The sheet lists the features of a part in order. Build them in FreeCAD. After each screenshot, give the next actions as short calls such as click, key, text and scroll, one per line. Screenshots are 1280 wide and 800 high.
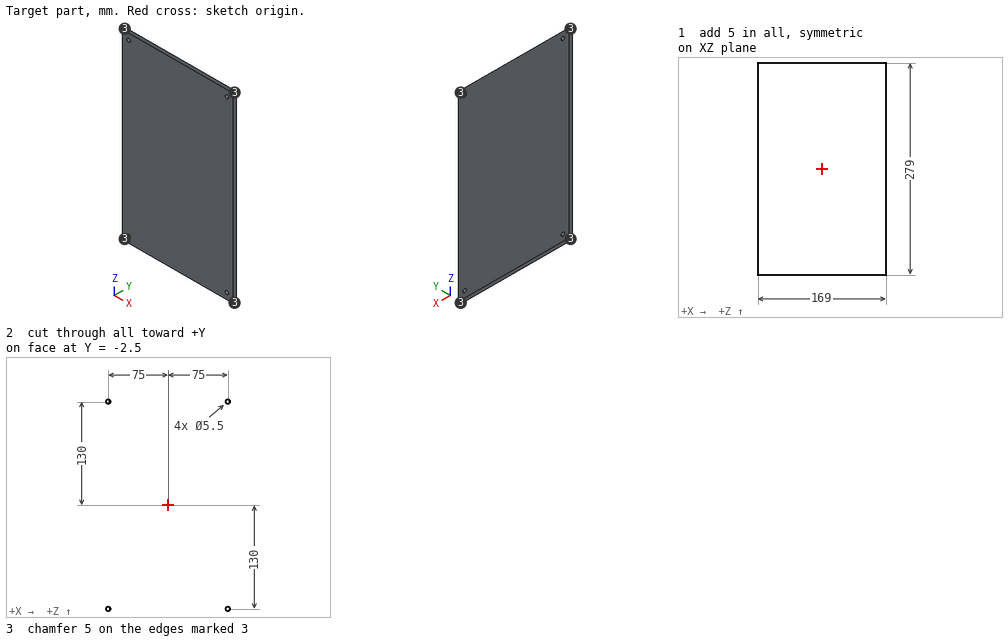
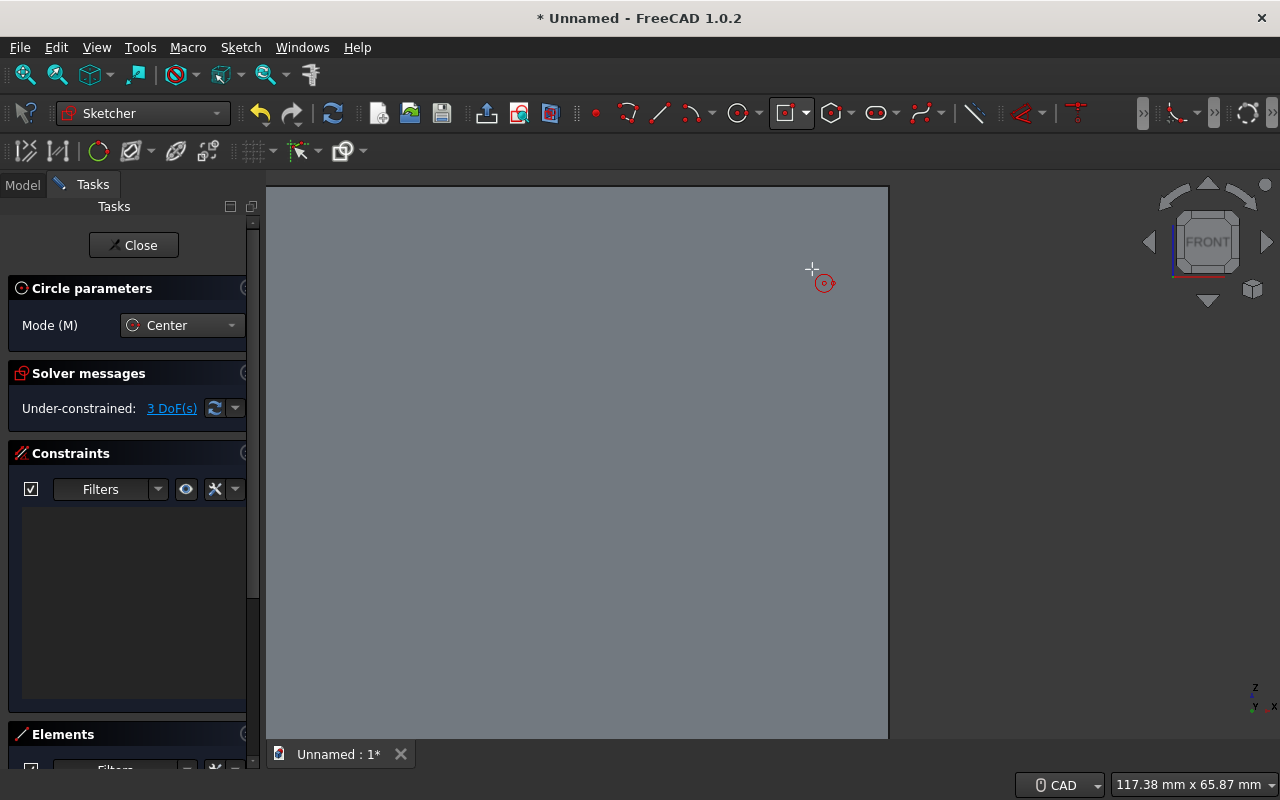
scroll(813, 269, down, 9)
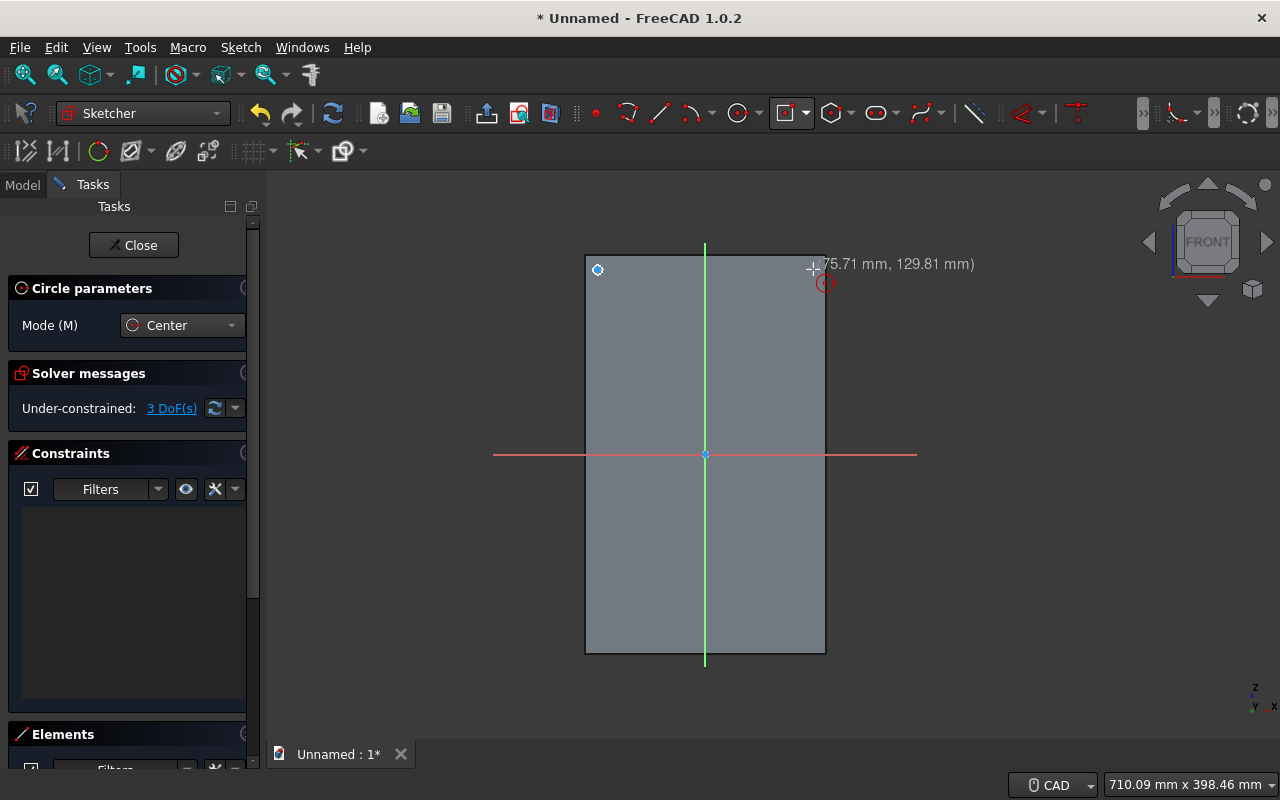
click(812, 269)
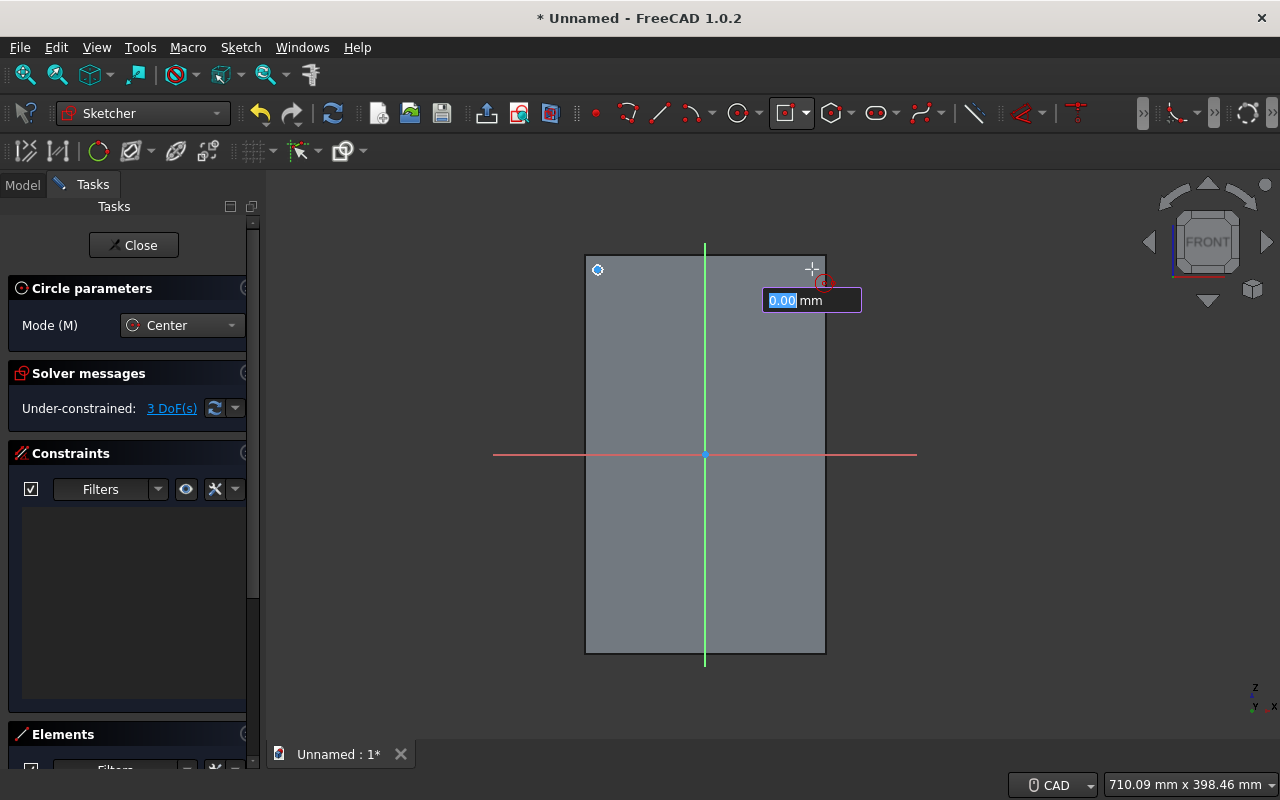
scroll(815, 266, up, 7)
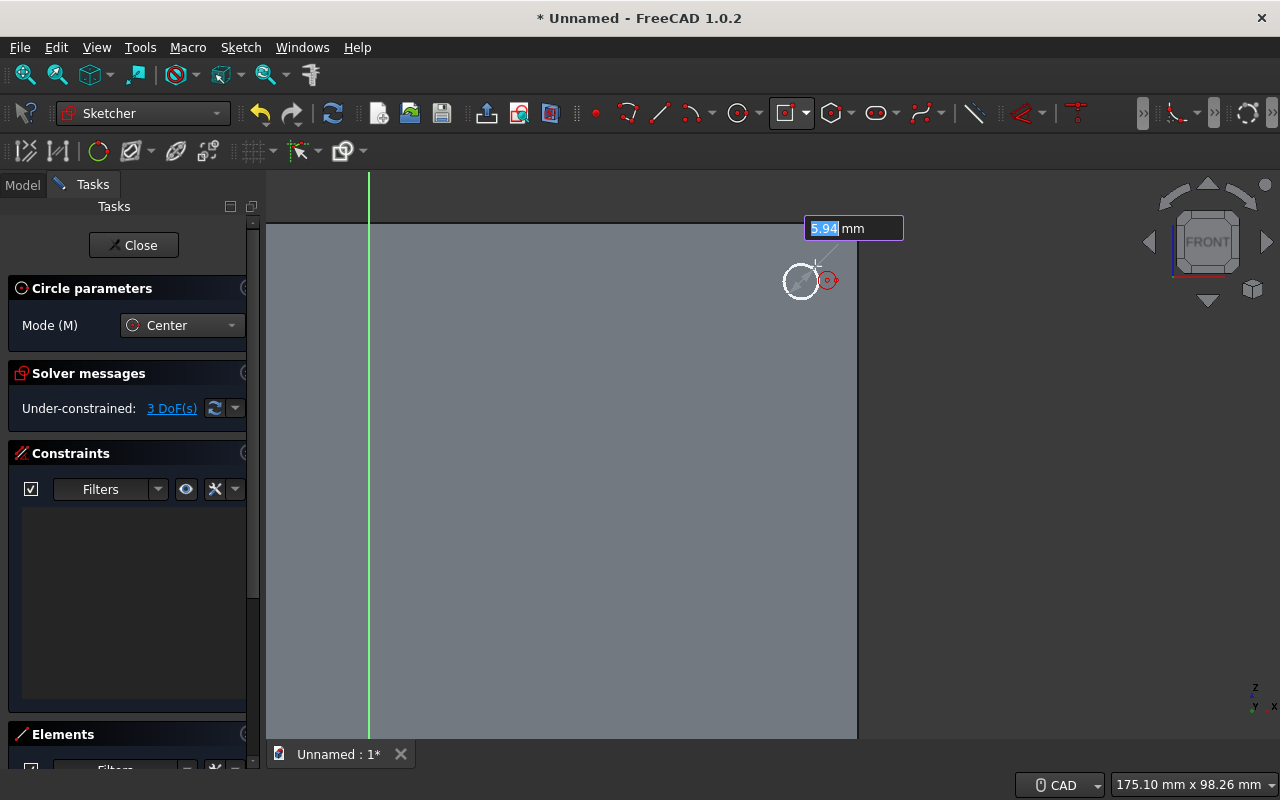
click(814, 267)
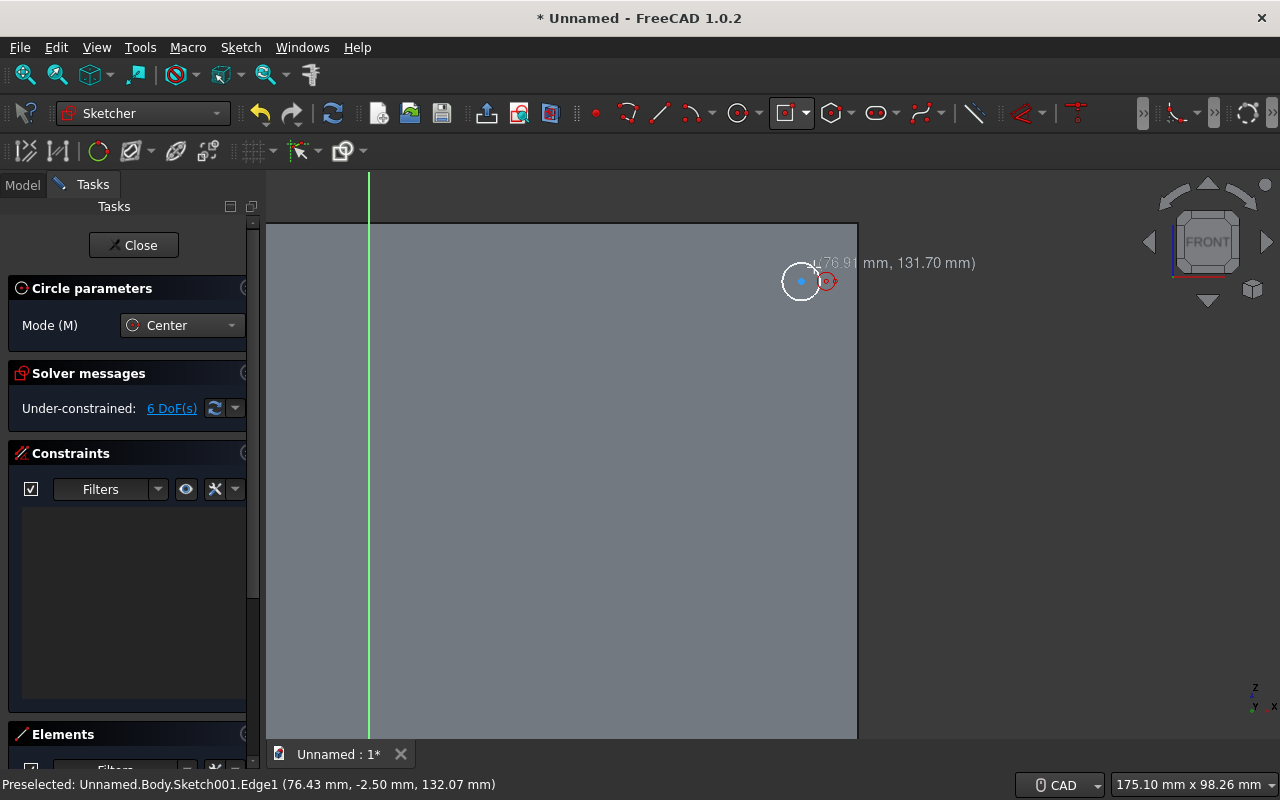
scroll(814, 266, down, 7)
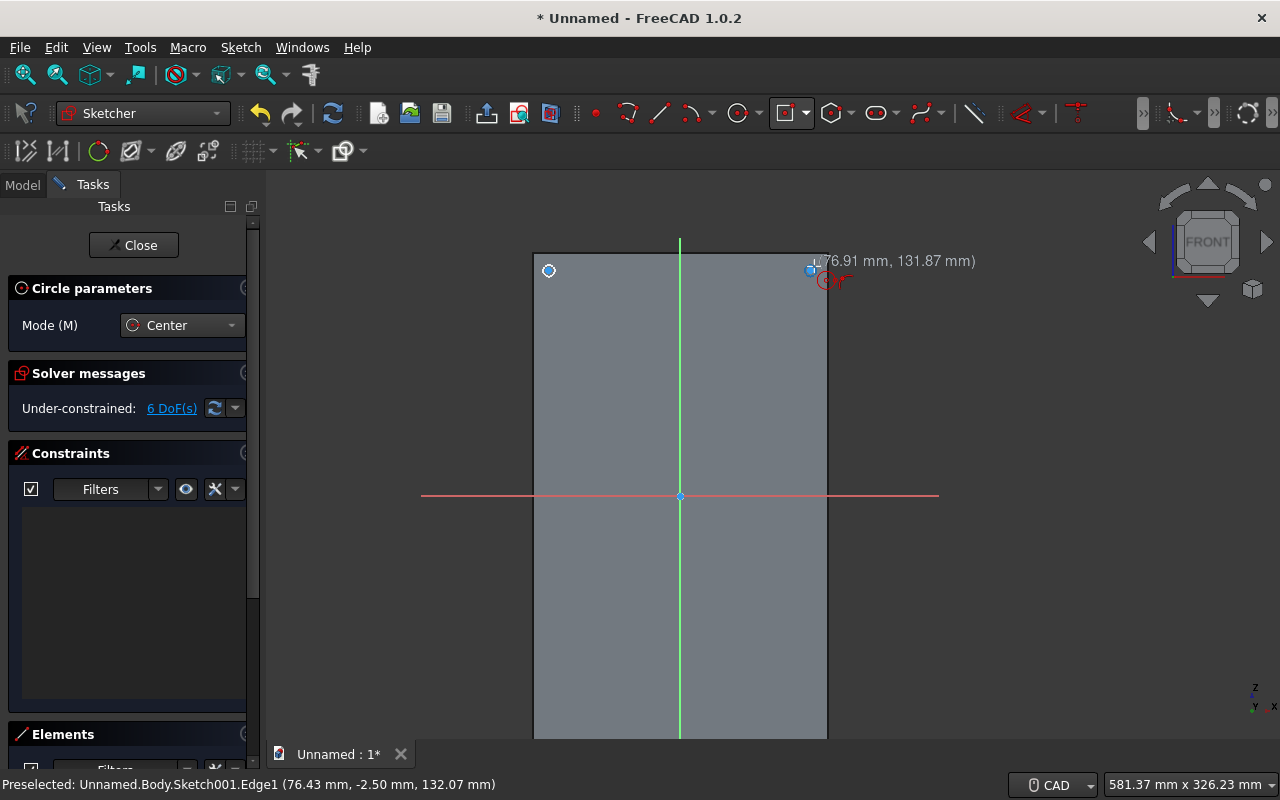
scroll(812, 640, up, 9)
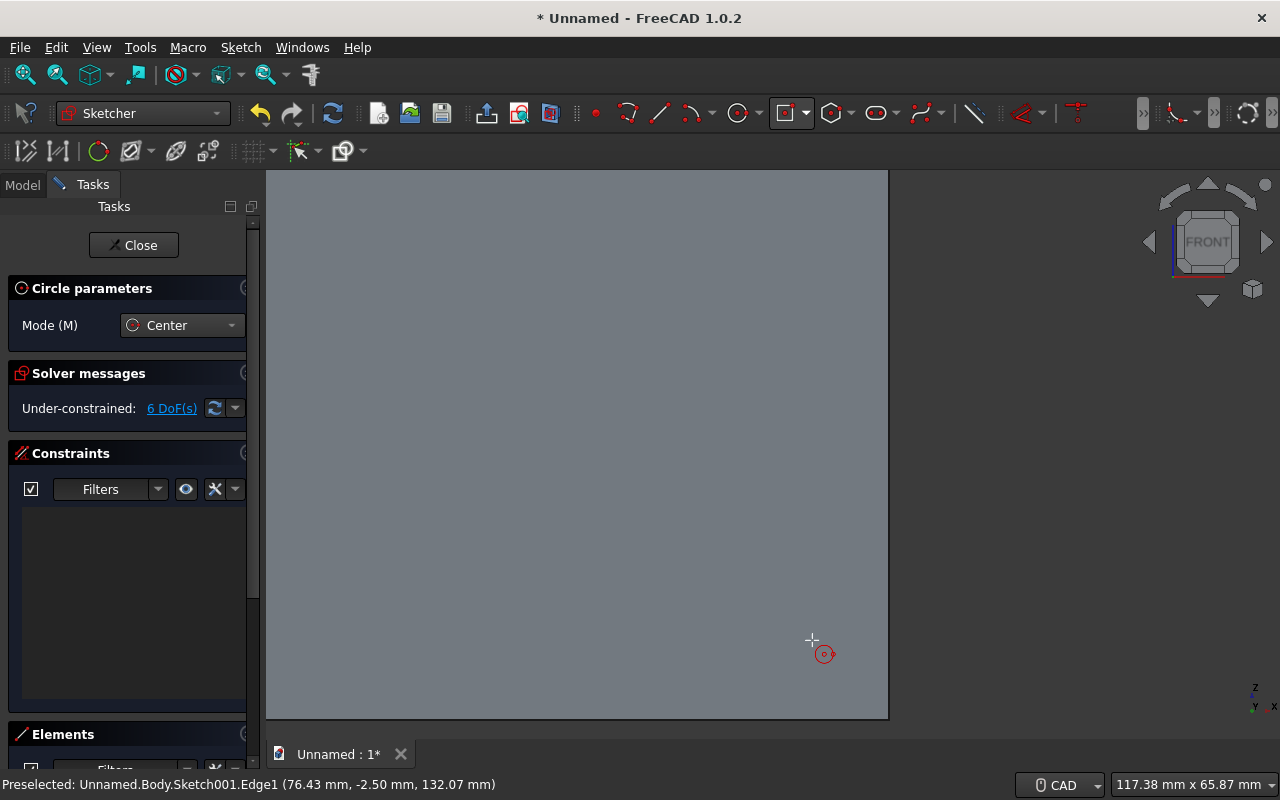
scroll(812, 641, down, 9)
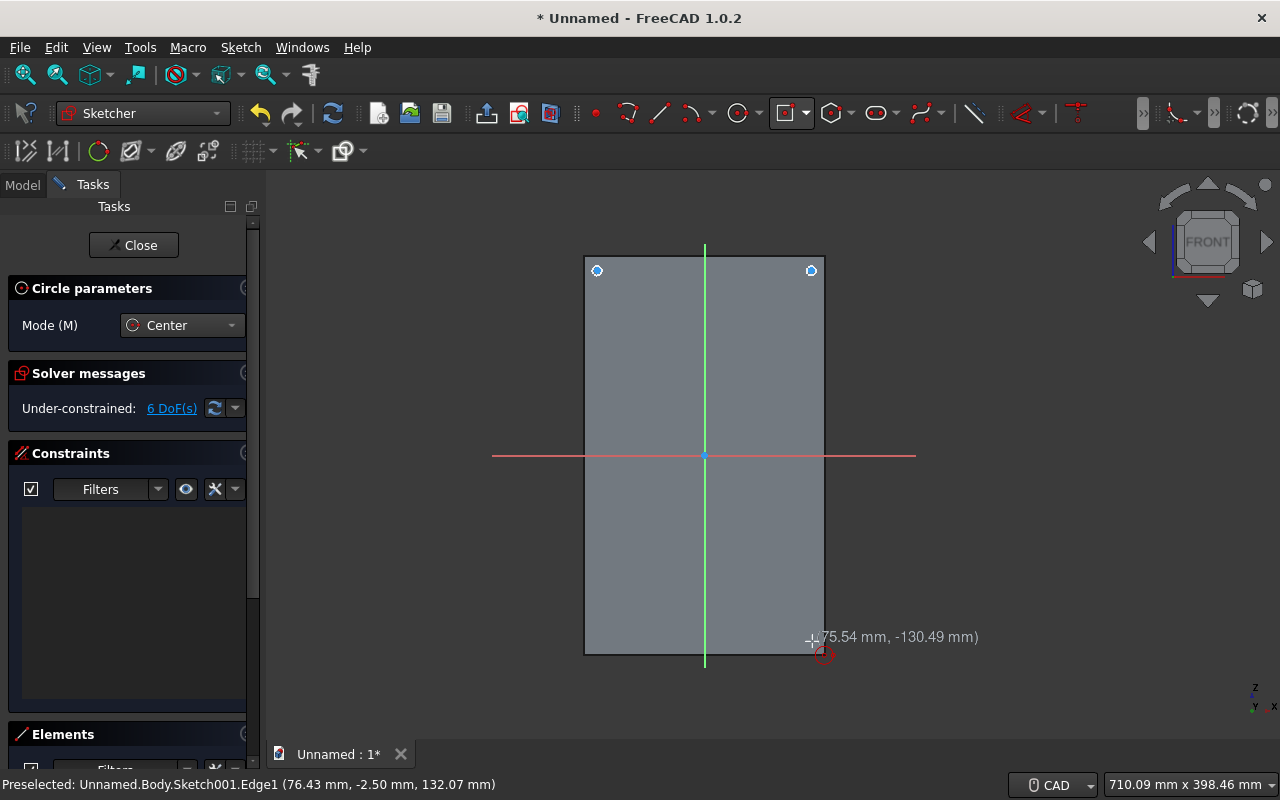
click(812, 641)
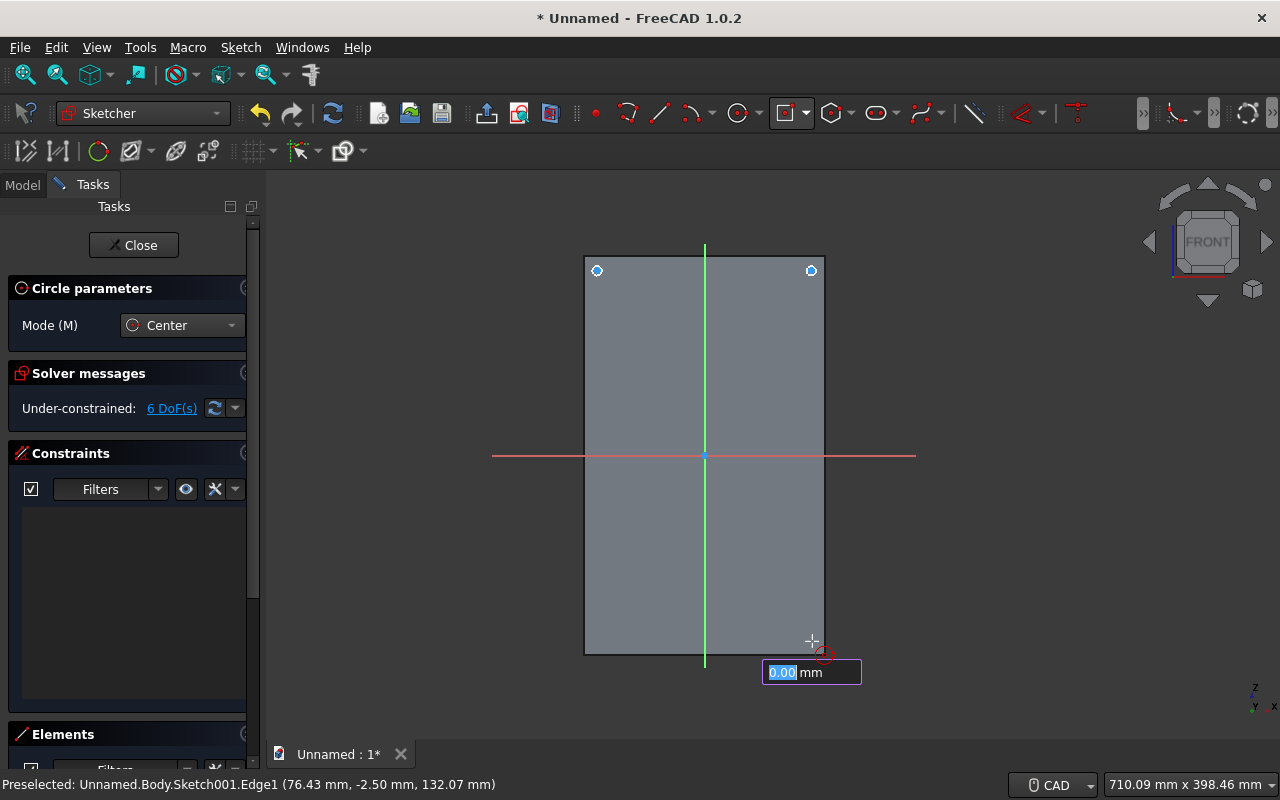
scroll(814, 638, up, 7)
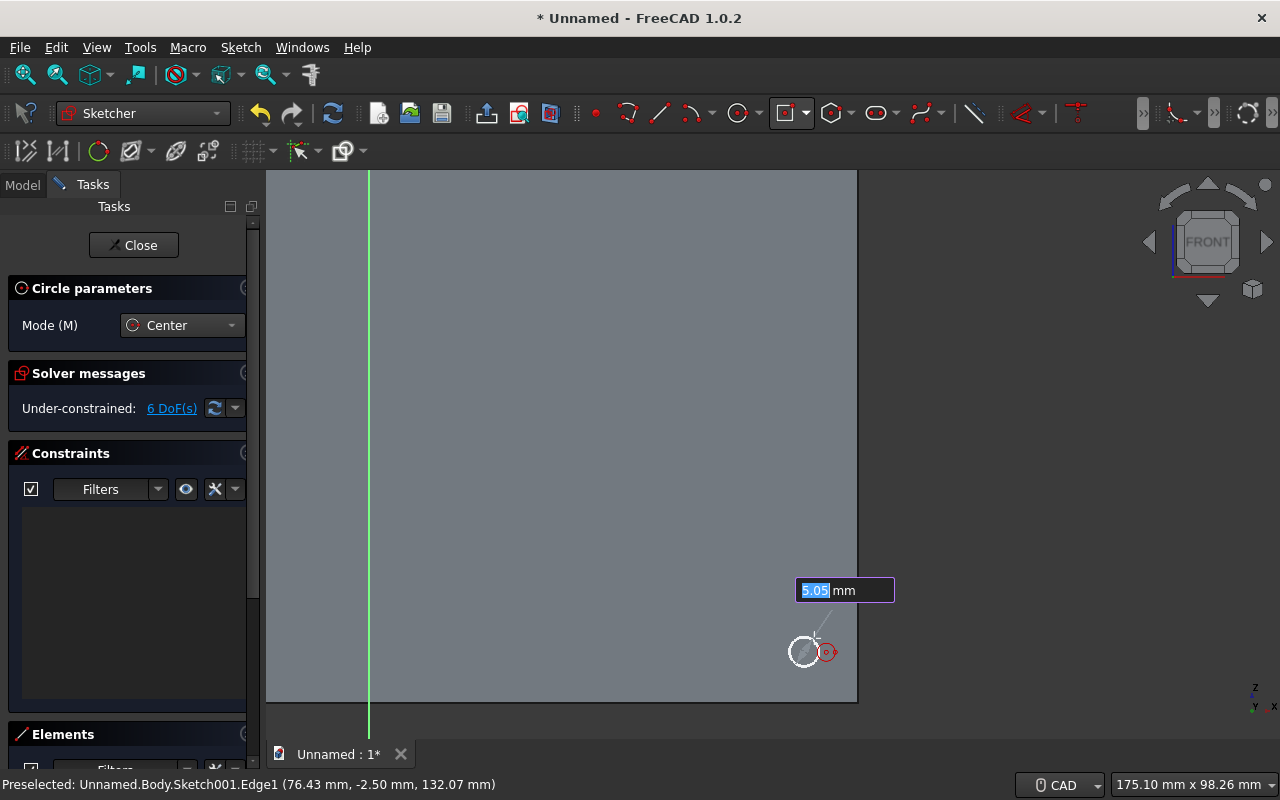
click(814, 637)